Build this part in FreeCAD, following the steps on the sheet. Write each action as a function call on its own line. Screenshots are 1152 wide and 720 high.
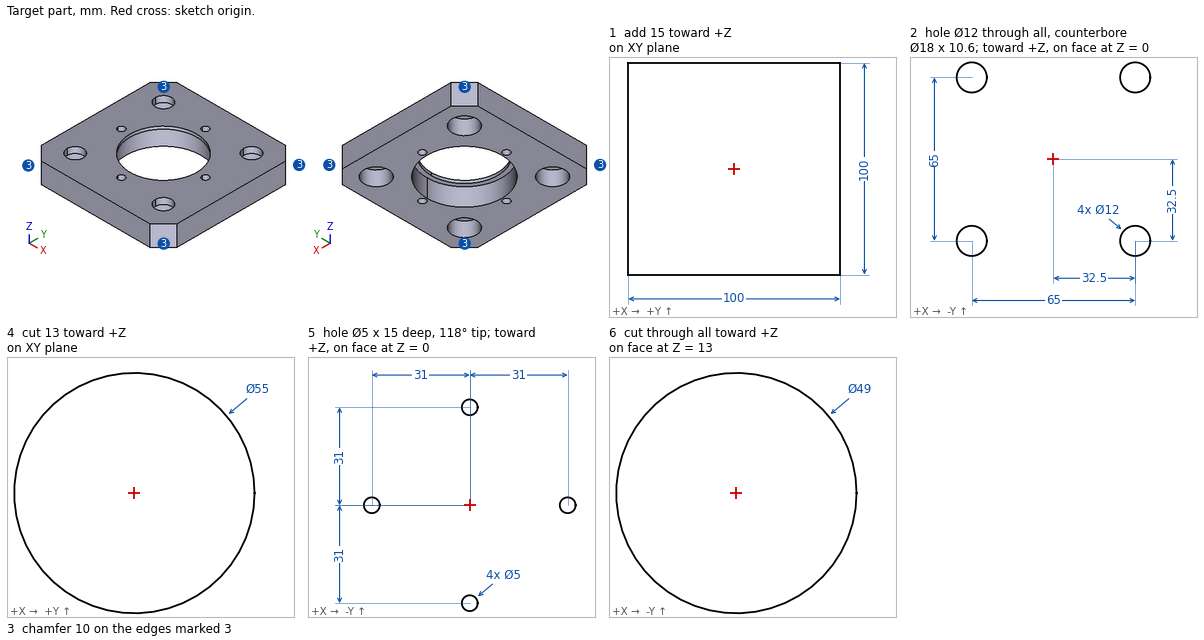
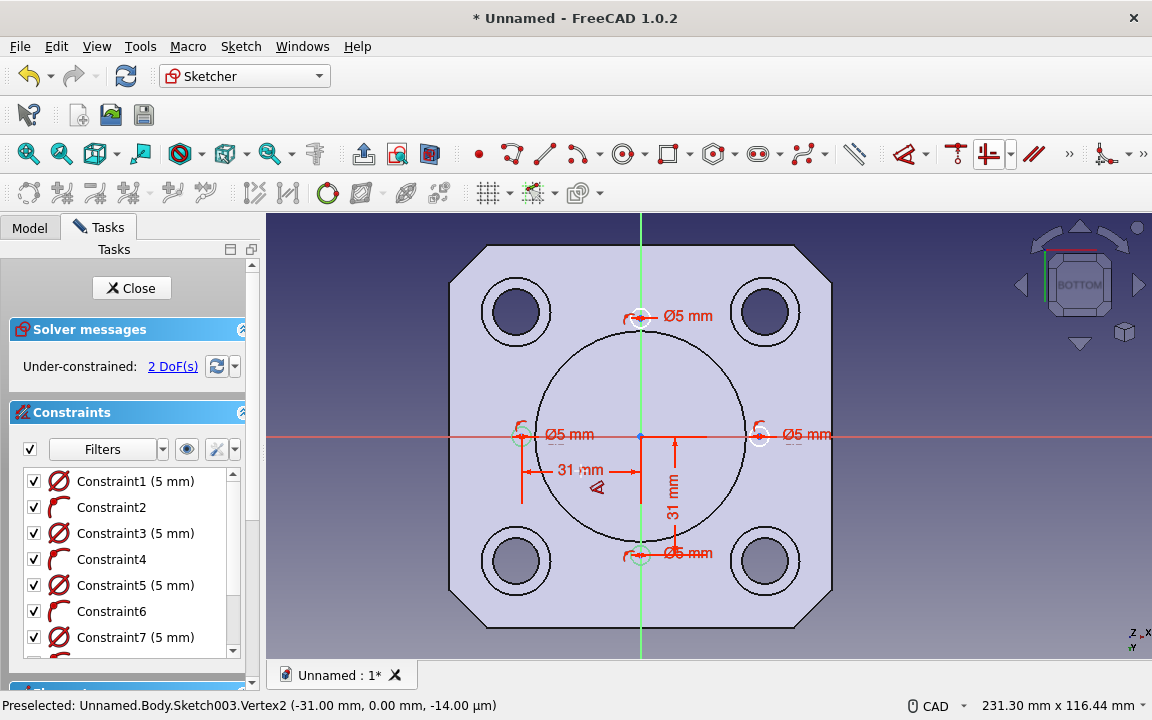
click(641, 318)
click(675, 377)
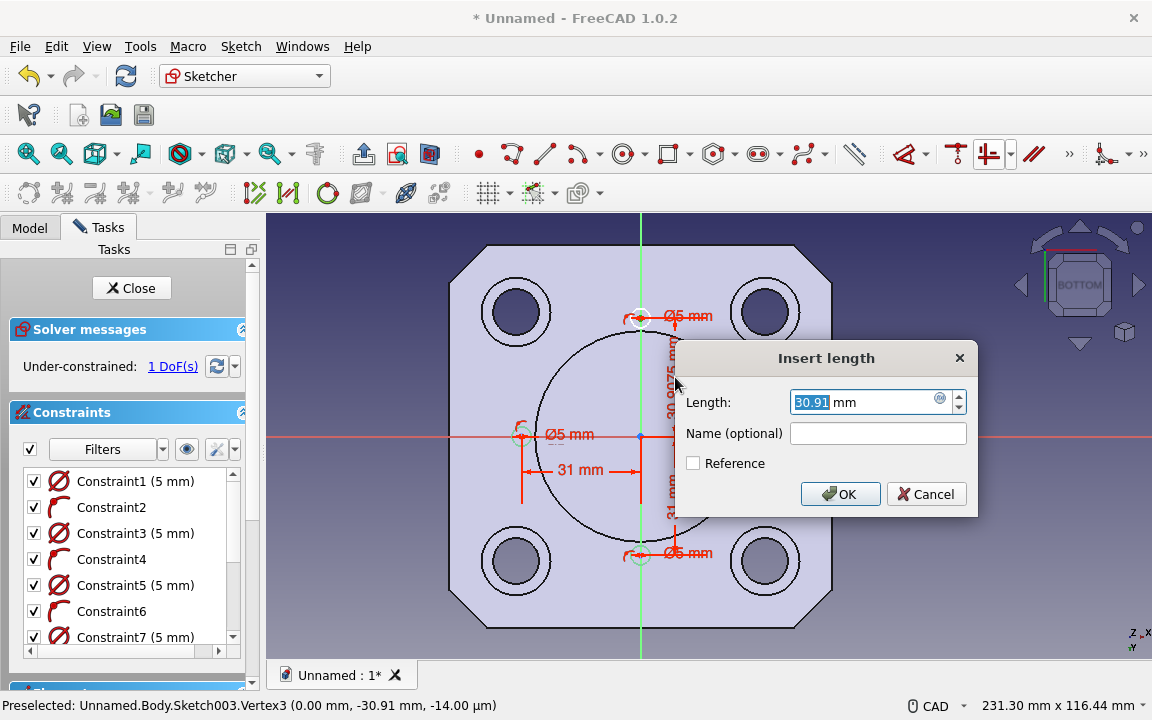
text(31)
key(Return)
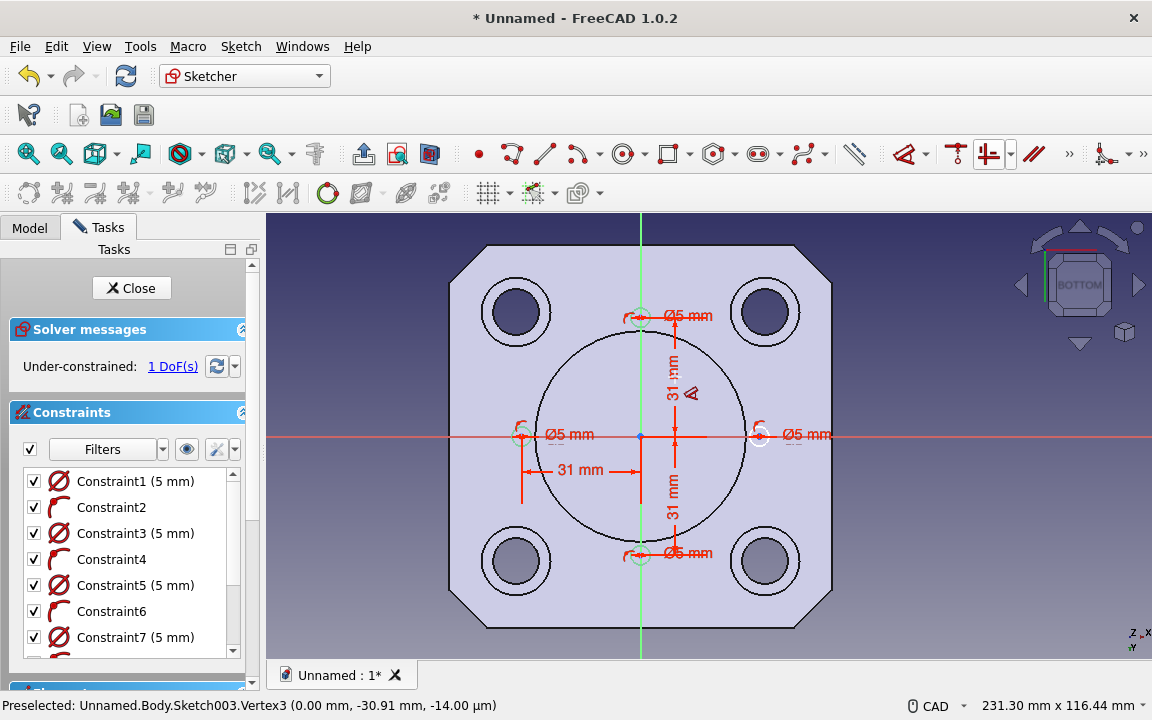
click(759, 437)
click(700, 471)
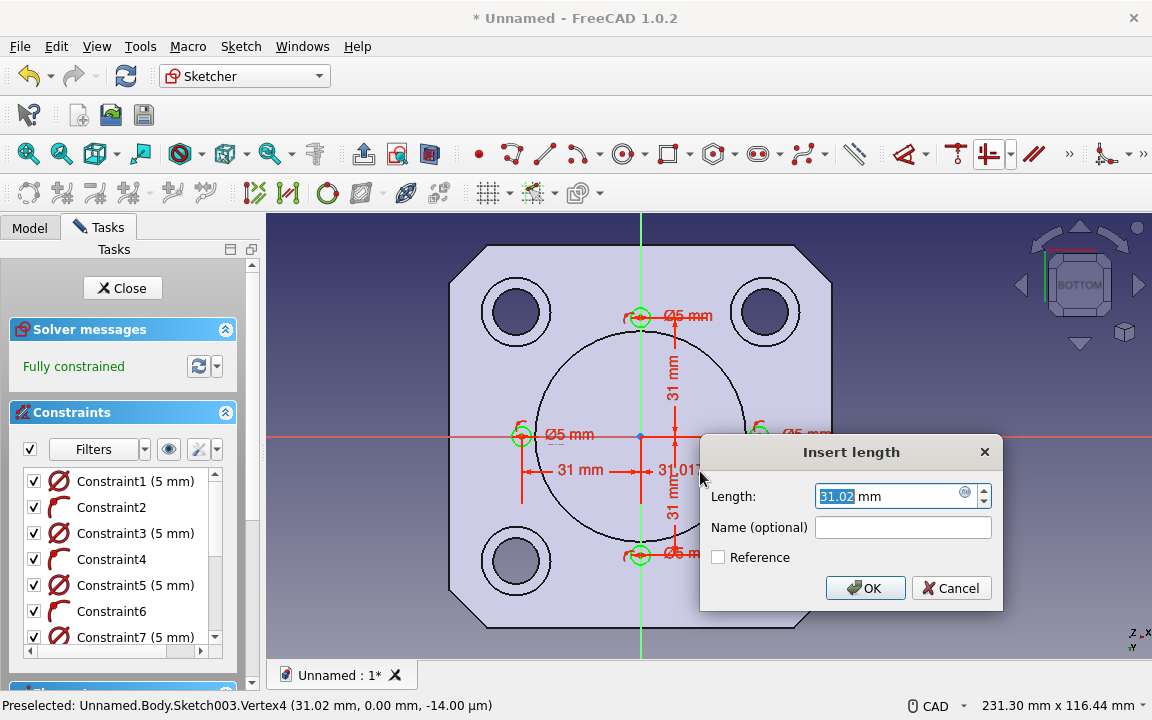
text(31)
key(Return)
key(Escape)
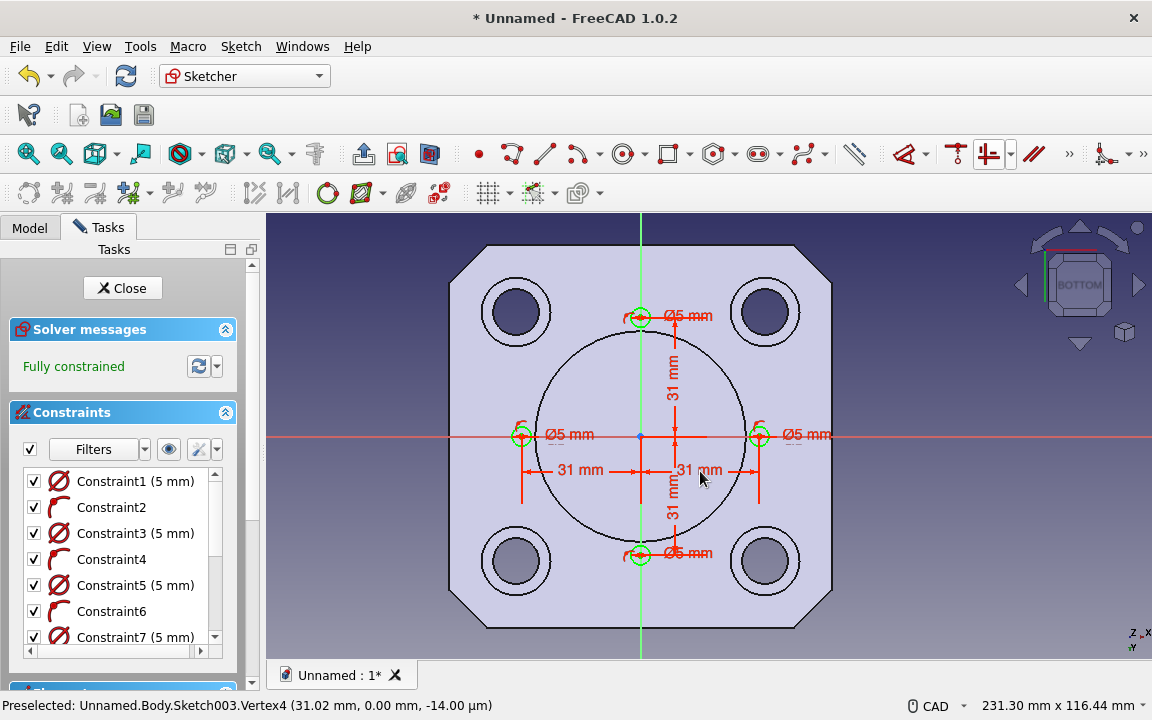
click(123, 288)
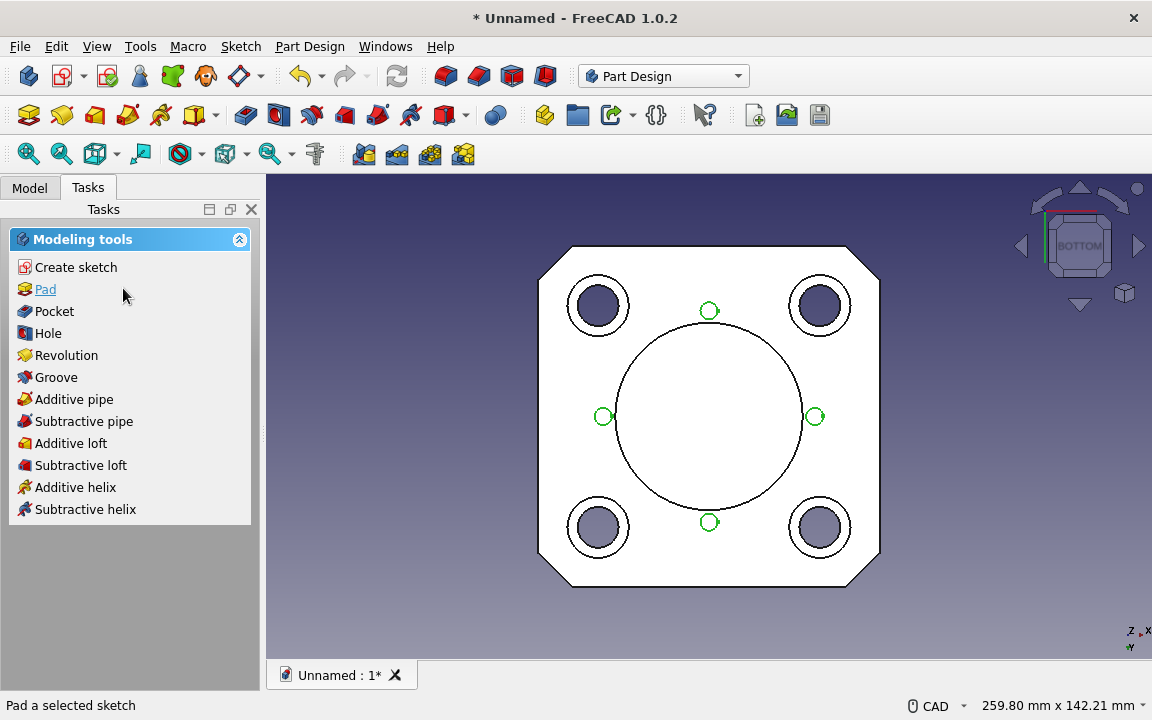
click(279, 116)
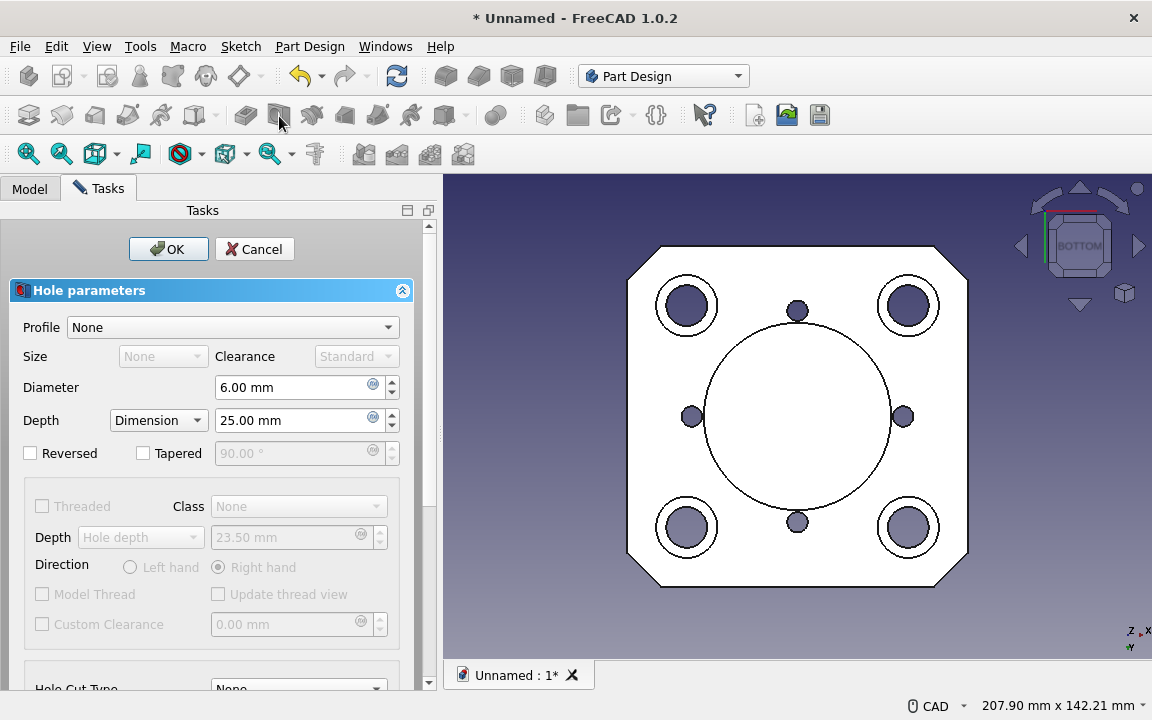
triple_click(300, 388)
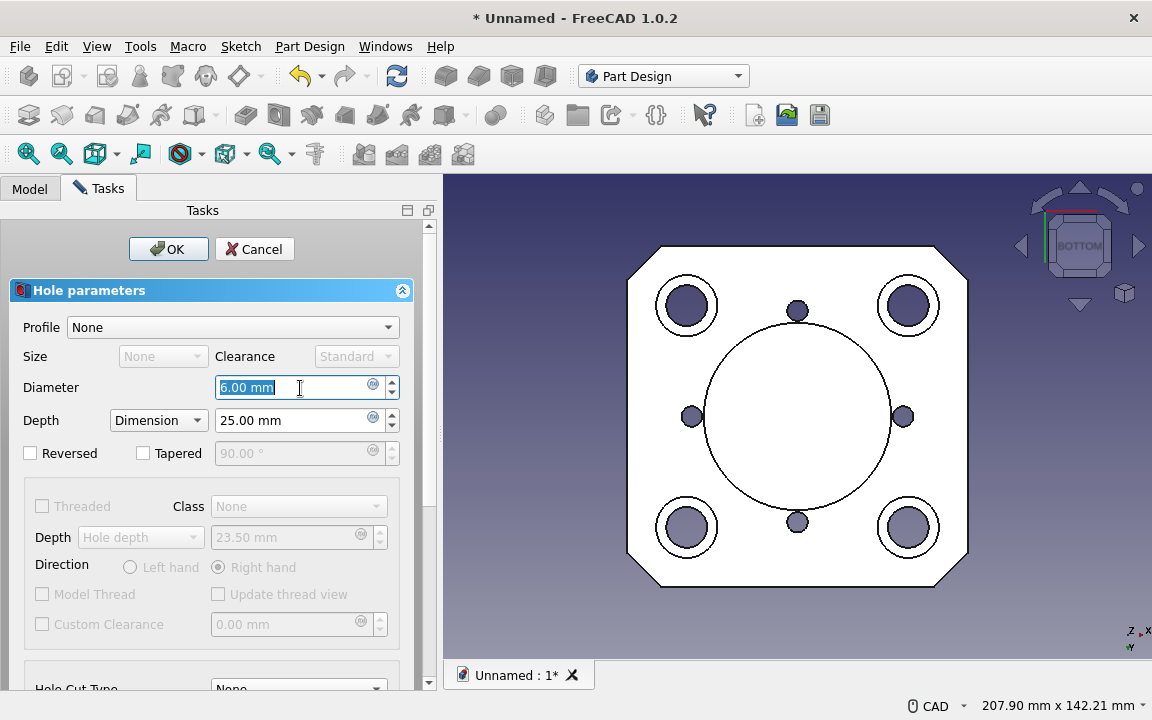
text(5)
key(Tab)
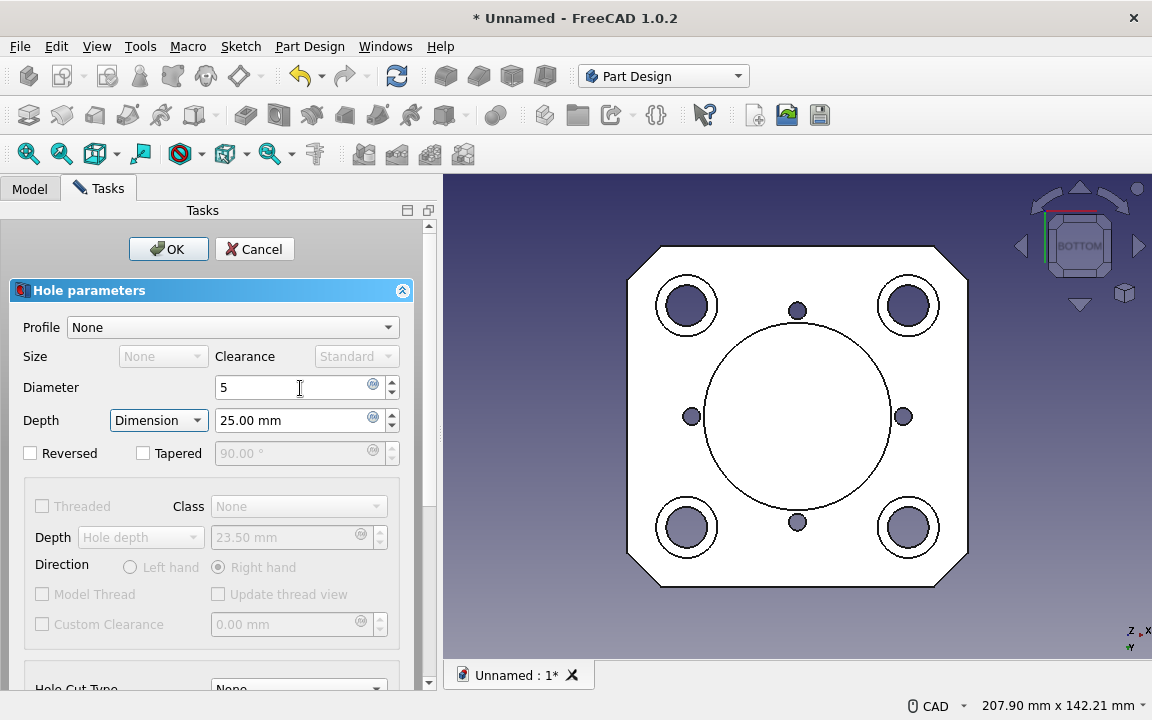
triple_click(300, 420)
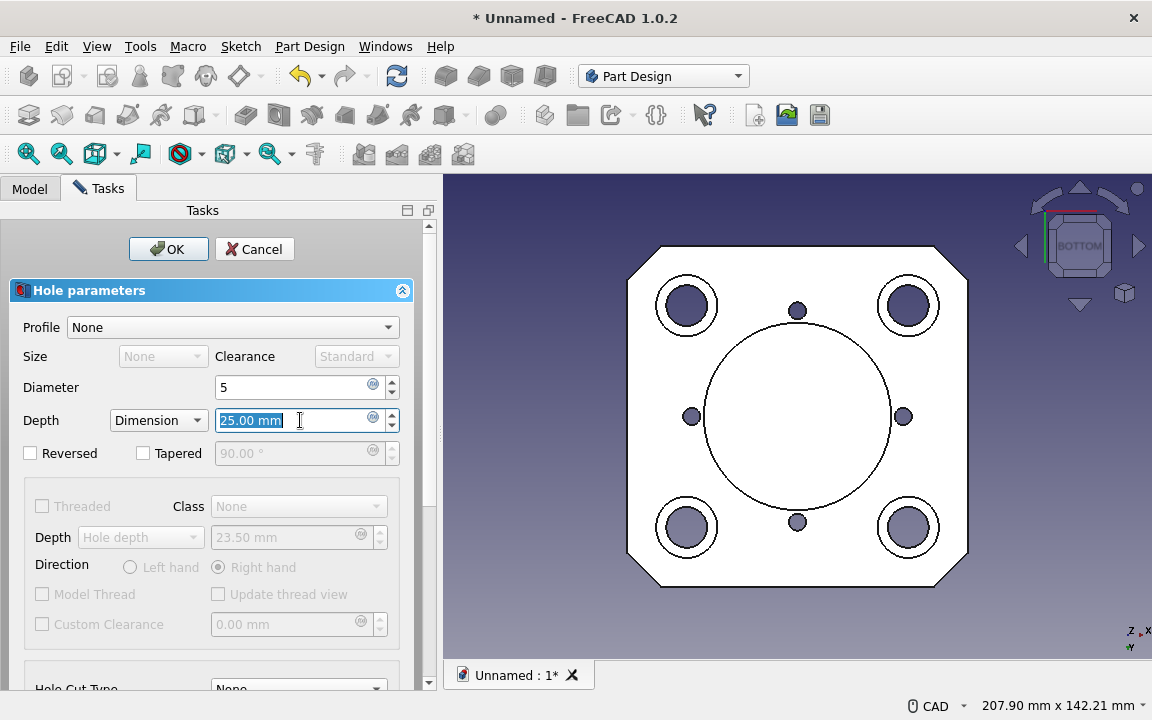
text(15)
key(Tab)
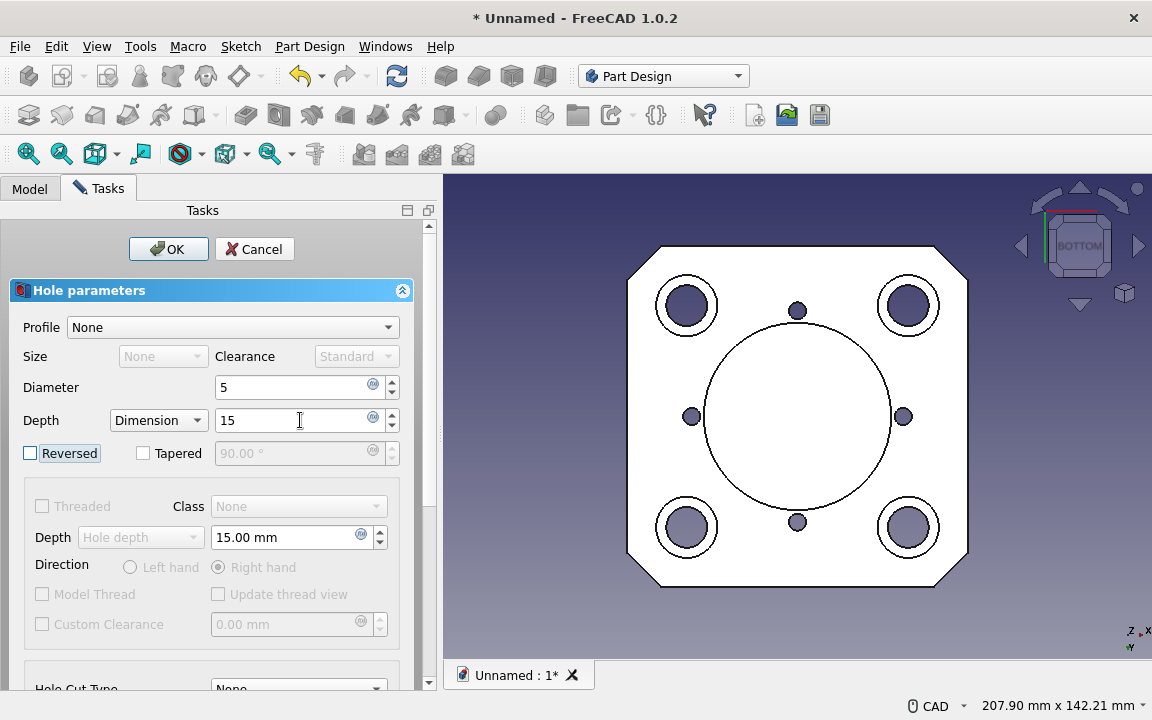
click(169, 249)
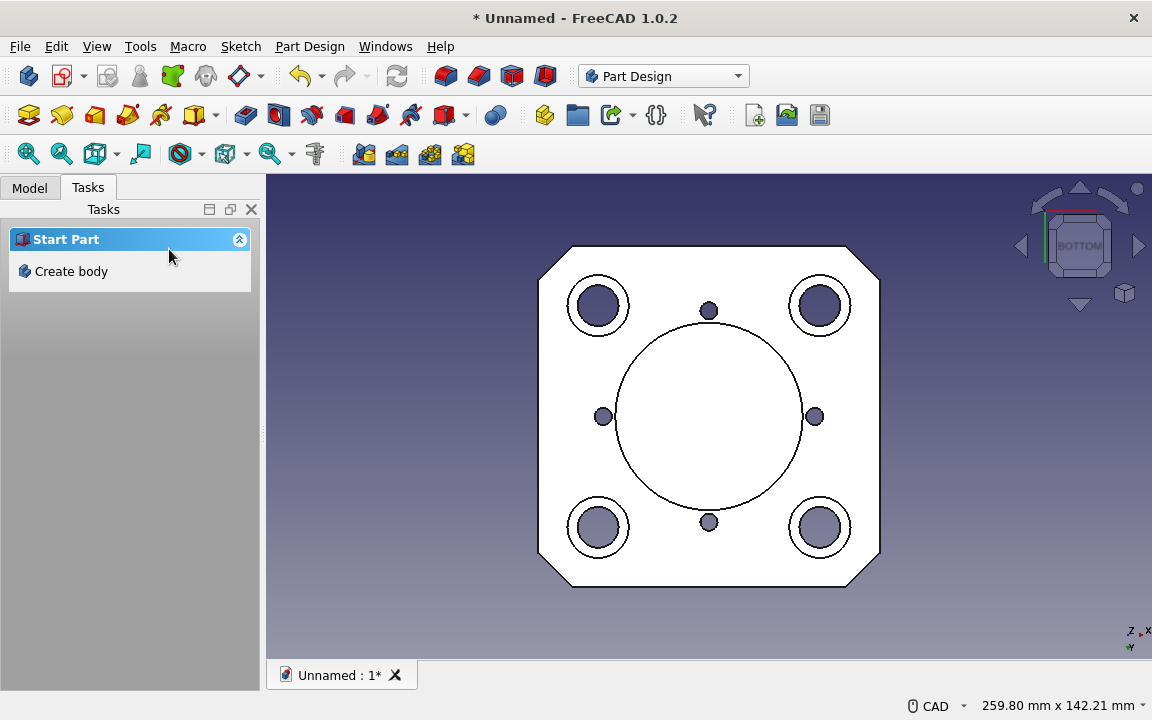
click(709, 416)